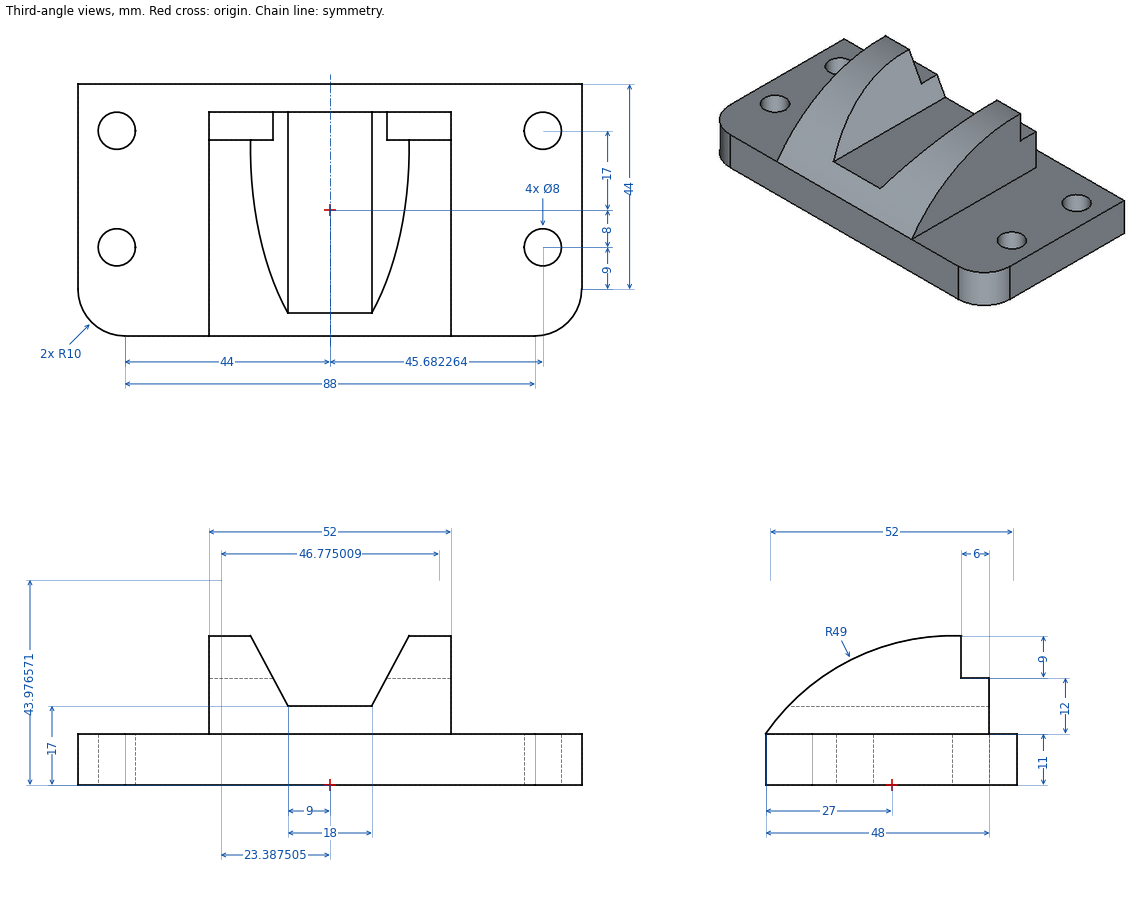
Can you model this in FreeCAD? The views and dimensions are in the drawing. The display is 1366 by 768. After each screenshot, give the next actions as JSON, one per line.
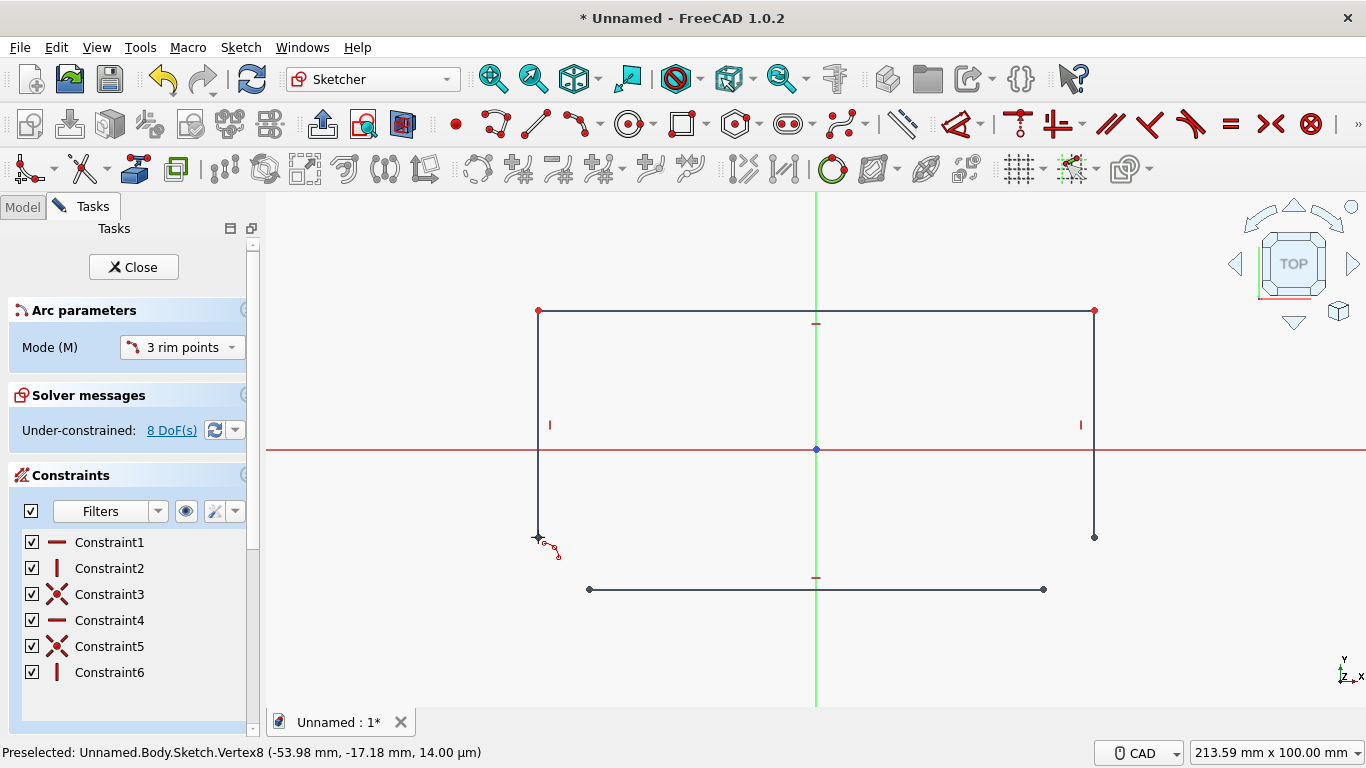
{"action": "left_click", "coordinate": [1043, 590]}
{"action": "left_click", "coordinate": [1094, 538]}
{"action": "left_click", "coordinate": [1079, 573]}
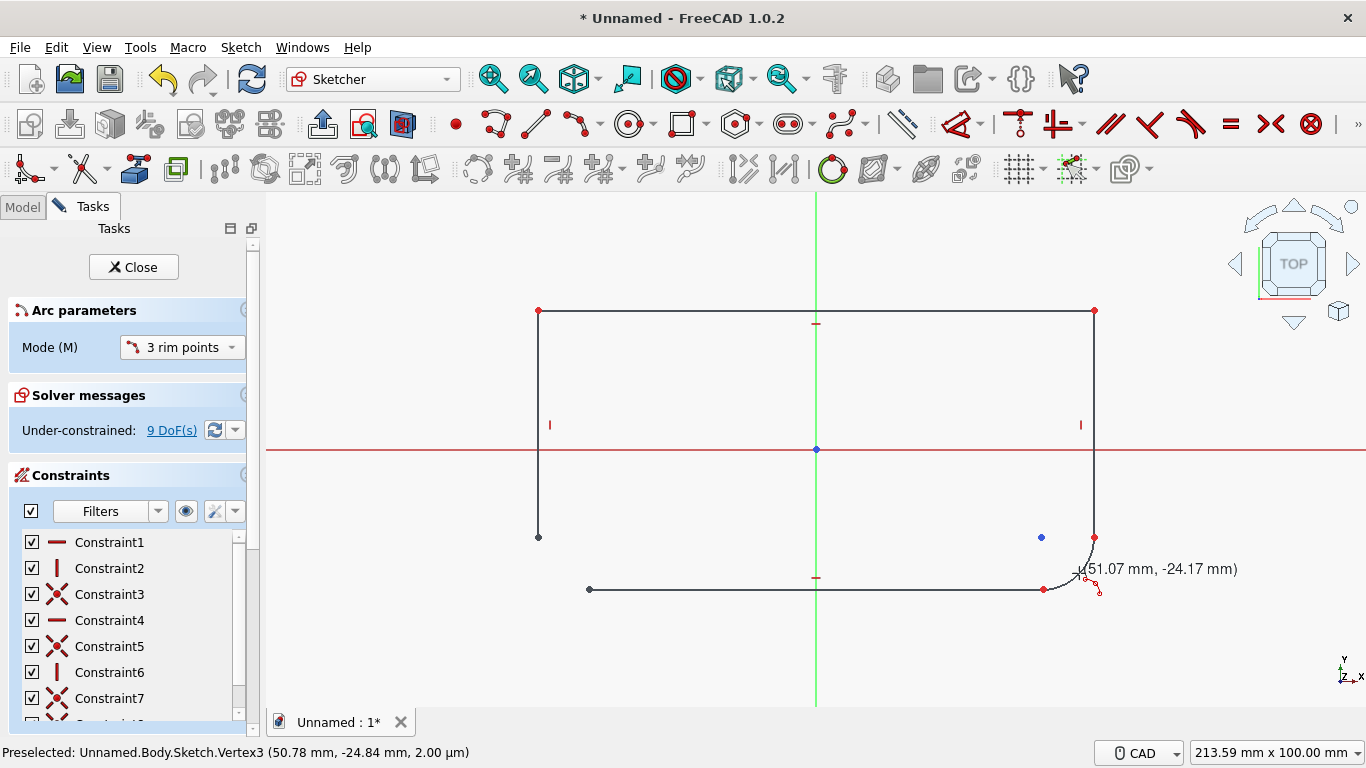
{"action": "left_click", "coordinate": [538, 538]}
{"action": "left_click", "coordinate": [589, 590]}
{"action": "left_click", "coordinate": [553, 573]}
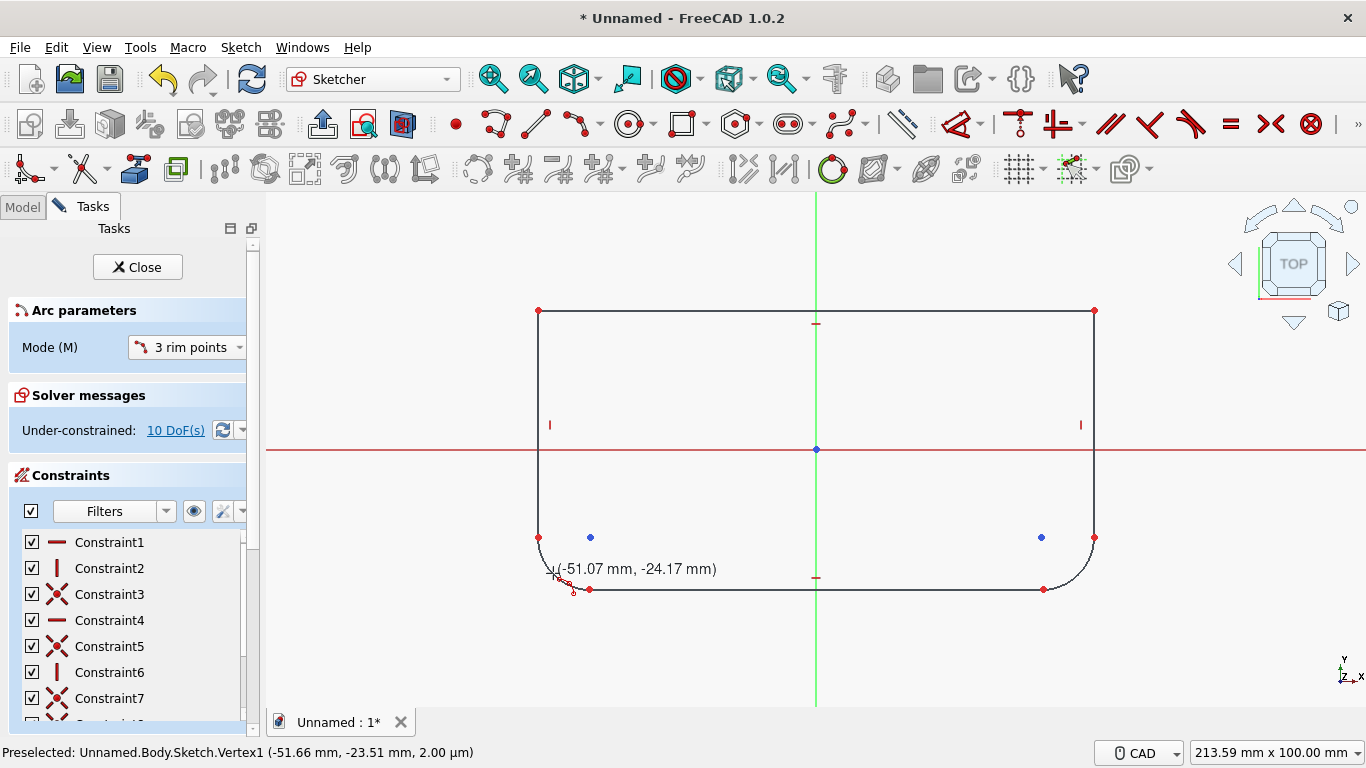
{"action": "key", "text": "g c"}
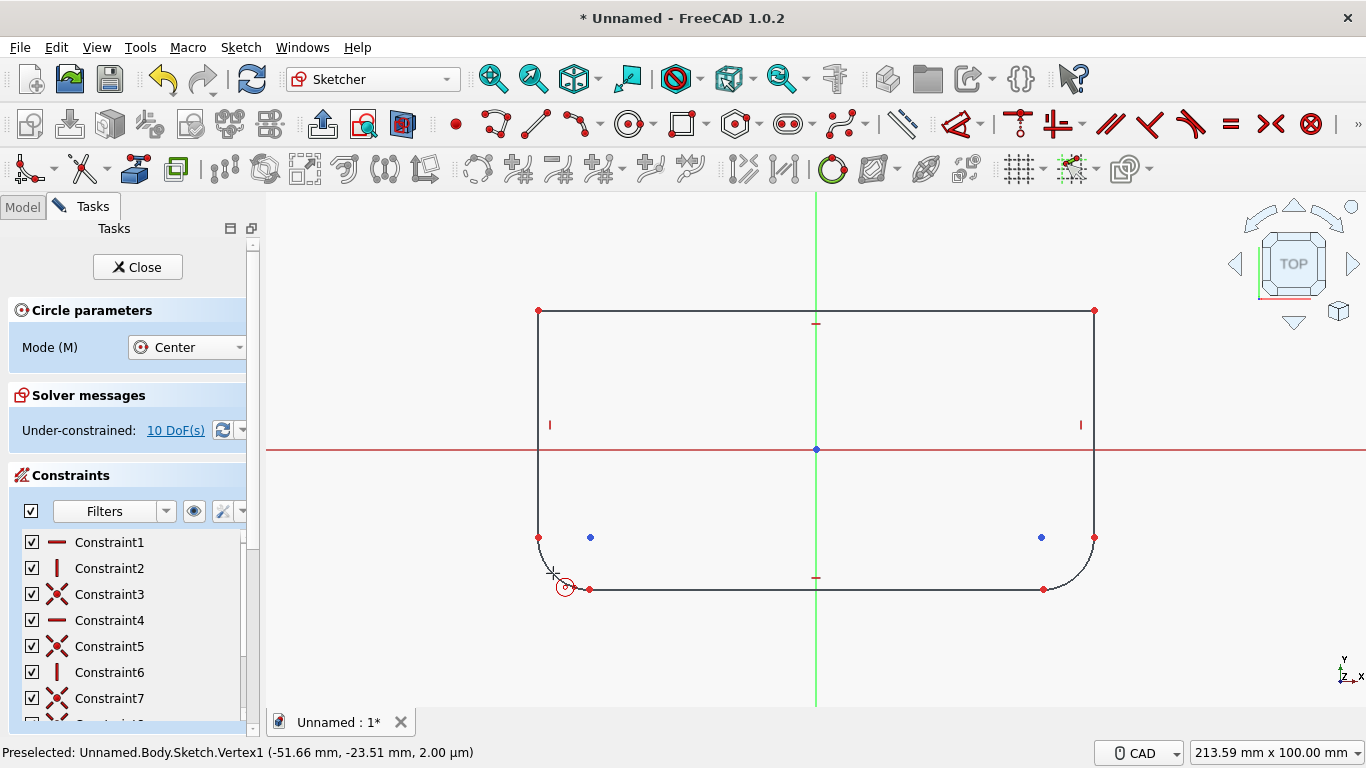
{"action": "left_click", "coordinate": [1051, 491]}
{"action": "left_click", "coordinate": [1066, 476]}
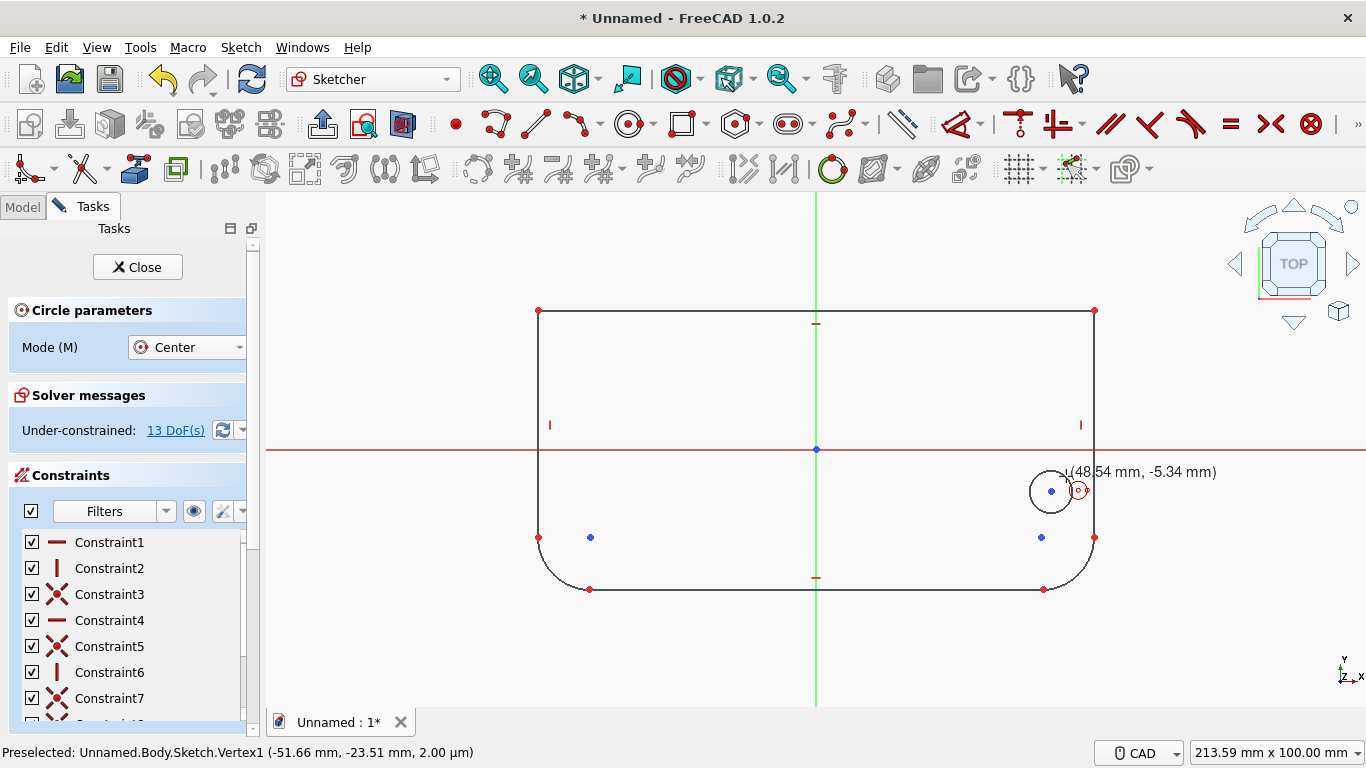
{"action": "left_click", "coordinate": [581, 491]}
{"action": "left_click", "coordinate": [595, 476]}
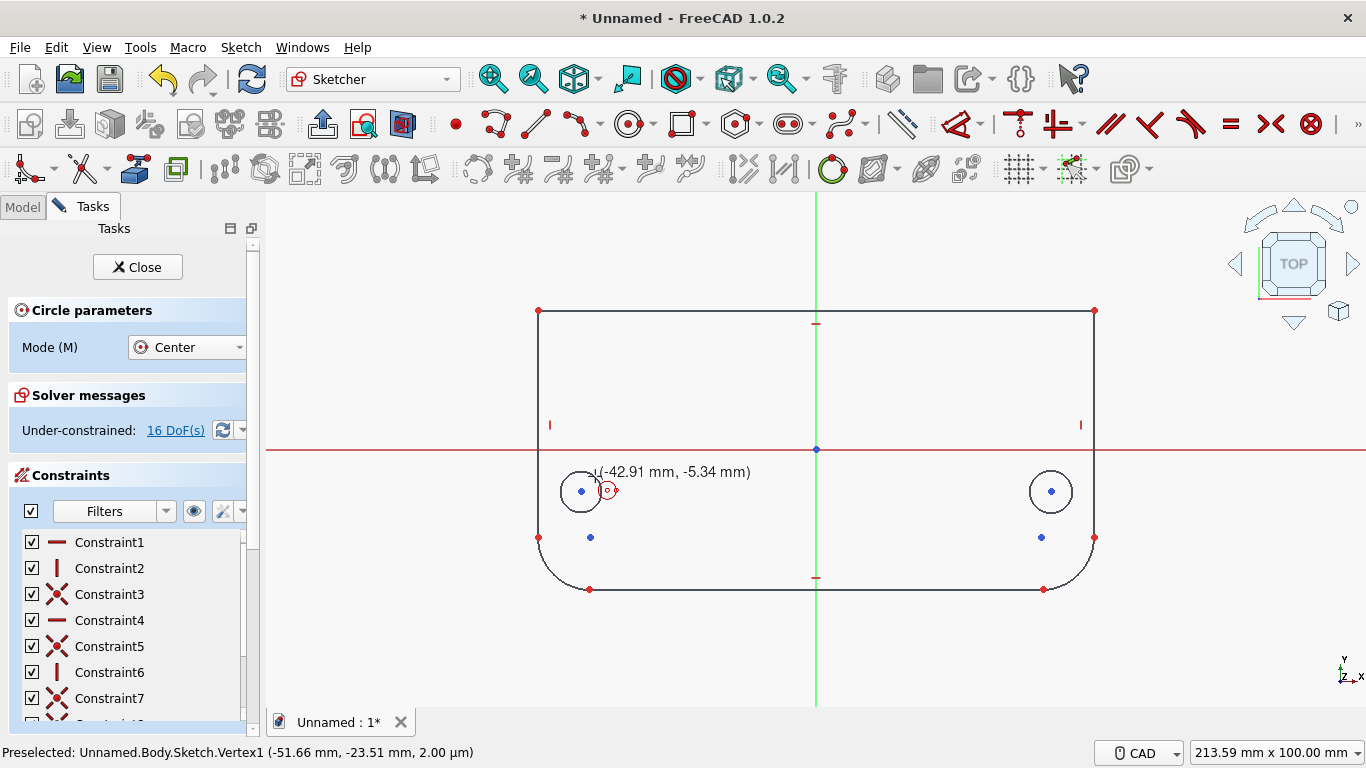
{"action": "left_click", "coordinate": [1051, 362]}
{"action": "left_click", "coordinate": [1066, 347]}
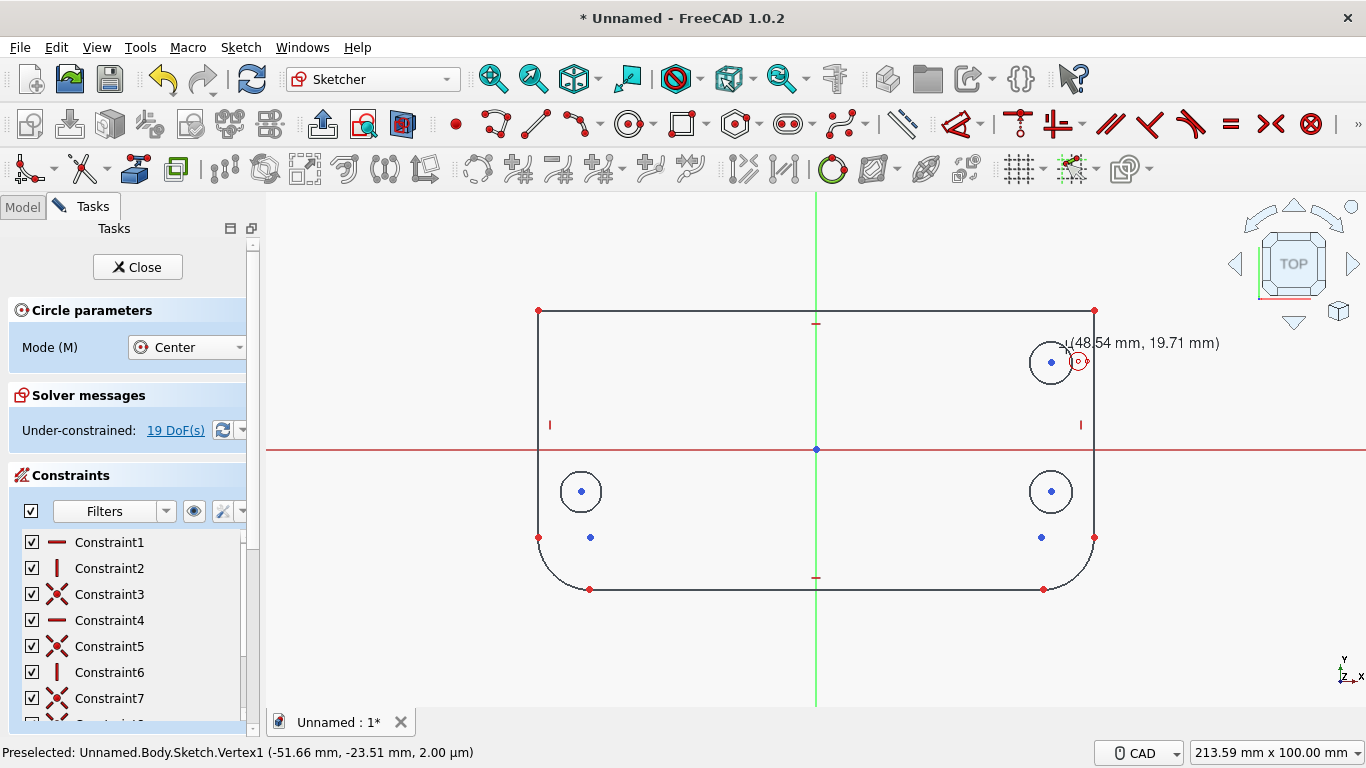
{"action": "left_click", "coordinate": [581, 362]}
{"action": "left_click", "coordinate": [595, 347]}
{"action": "key", "text": "Escape"}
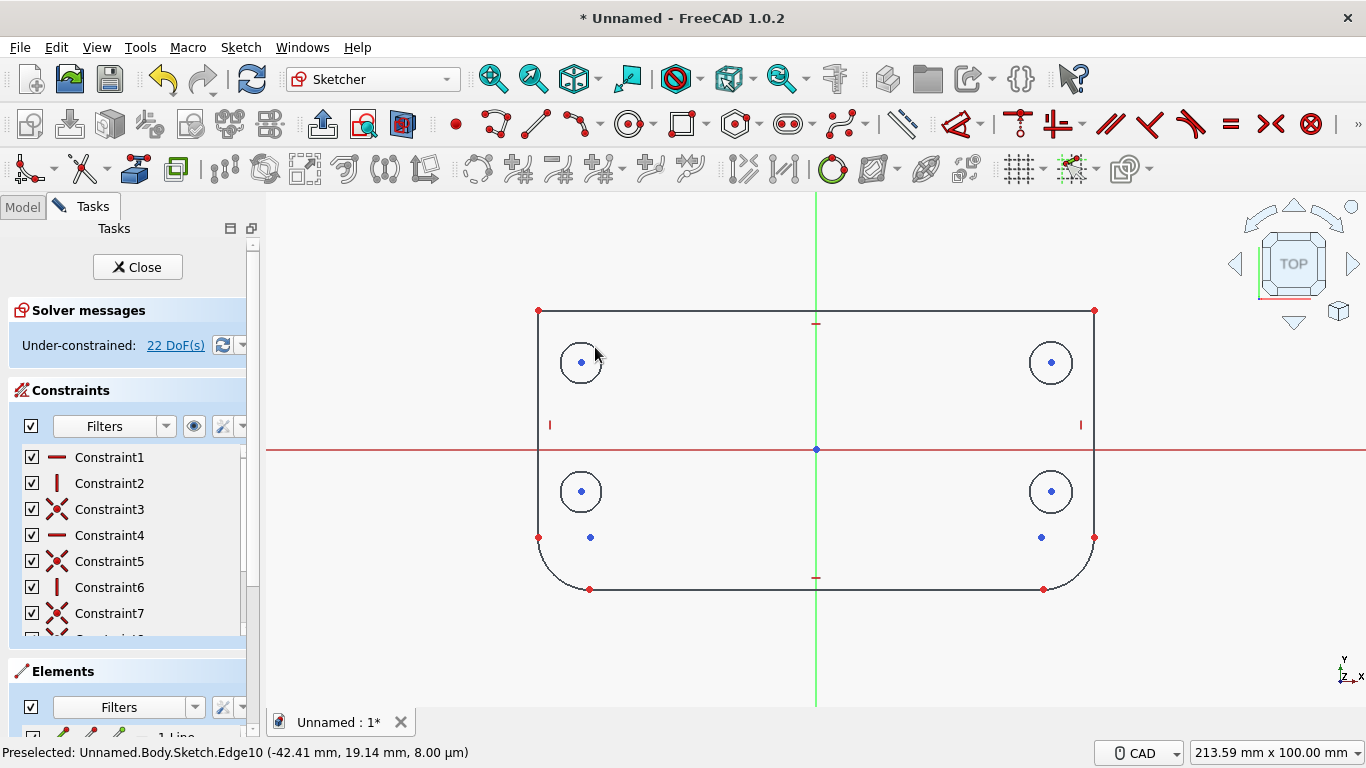
{"action": "left_click", "coordinate": [725, 590]}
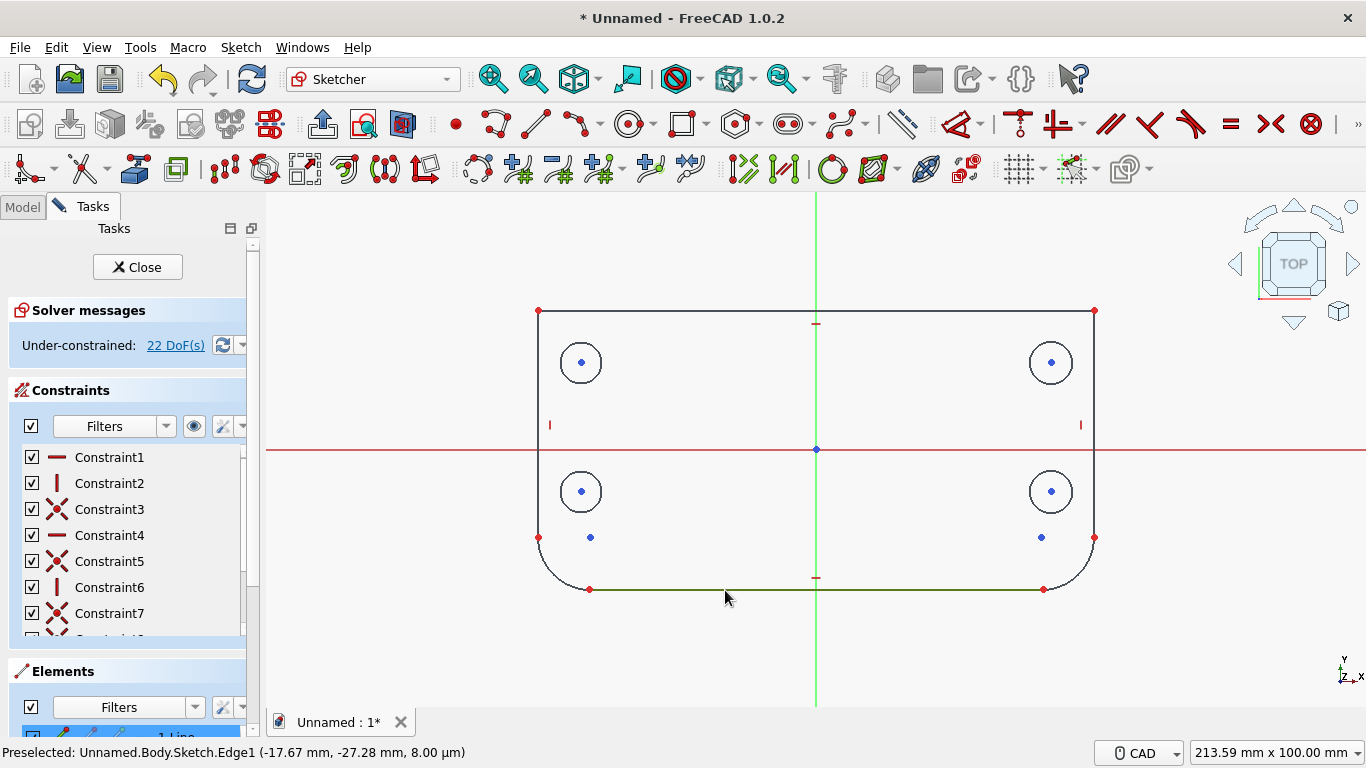
{"action": "left_click", "coordinate": [1066, 584]}